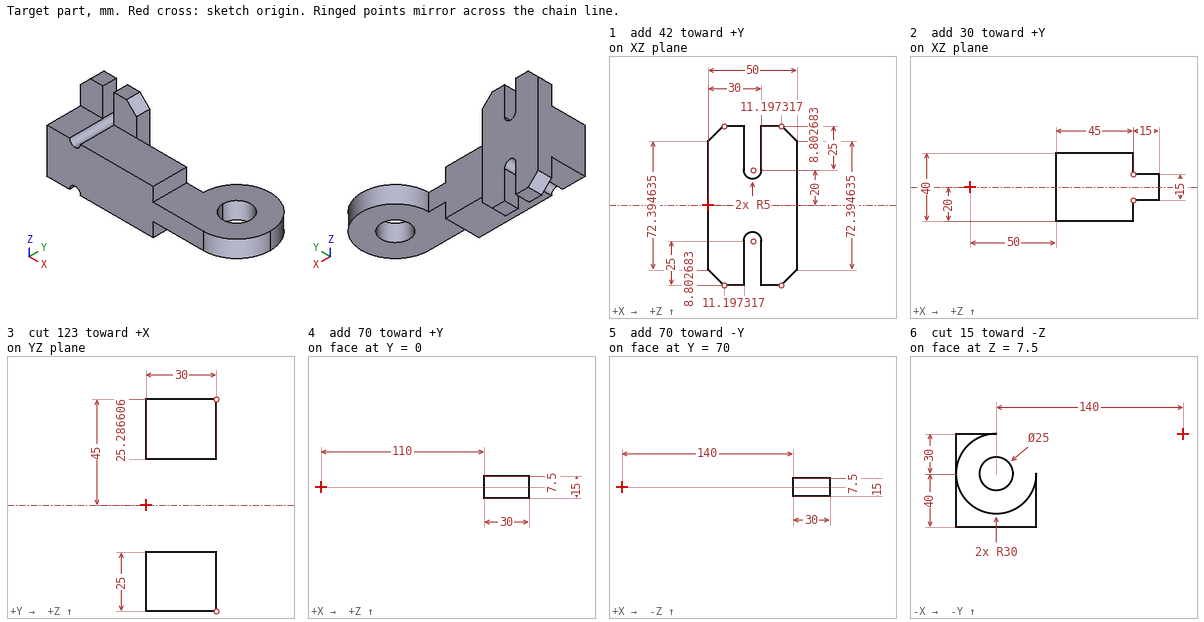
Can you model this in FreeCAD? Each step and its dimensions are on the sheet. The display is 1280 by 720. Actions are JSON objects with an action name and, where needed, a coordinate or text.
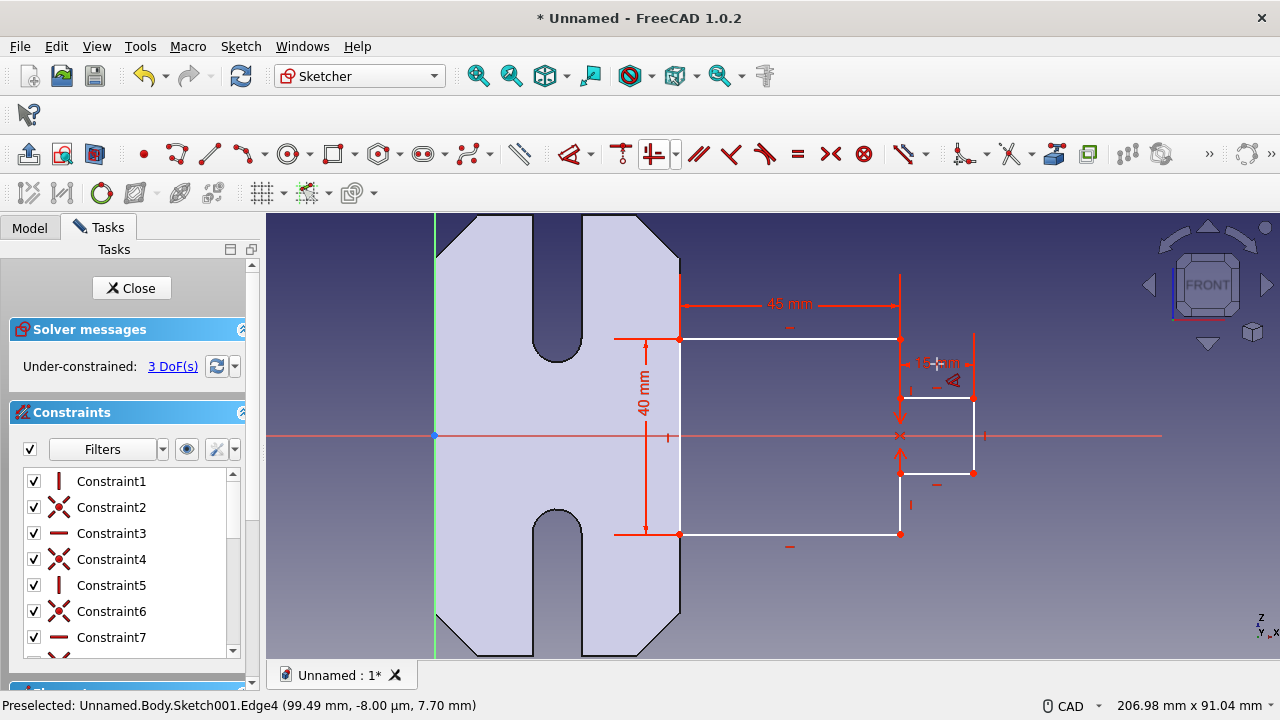
{"action": "left_click", "coordinate": [974, 421]}
{"action": "left_click", "coordinate": [1008, 419]}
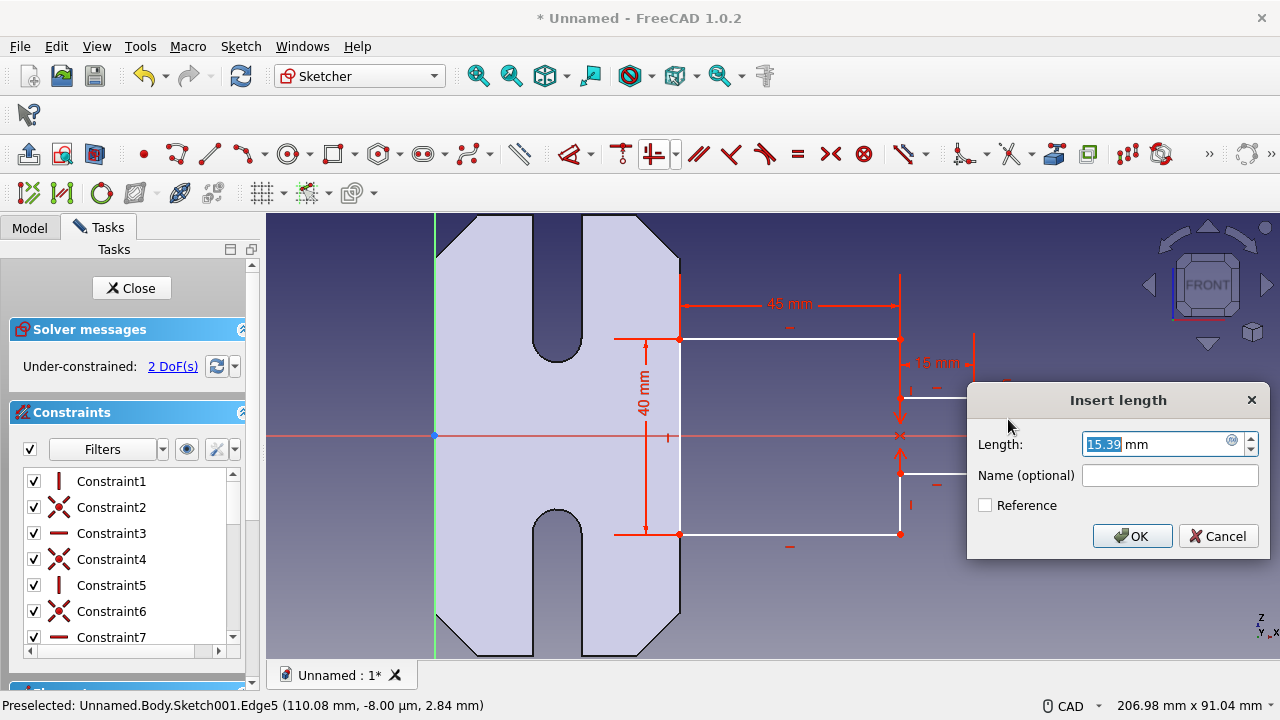
{"action": "type", "text": "15"}
{"action": "key", "text": "Return"}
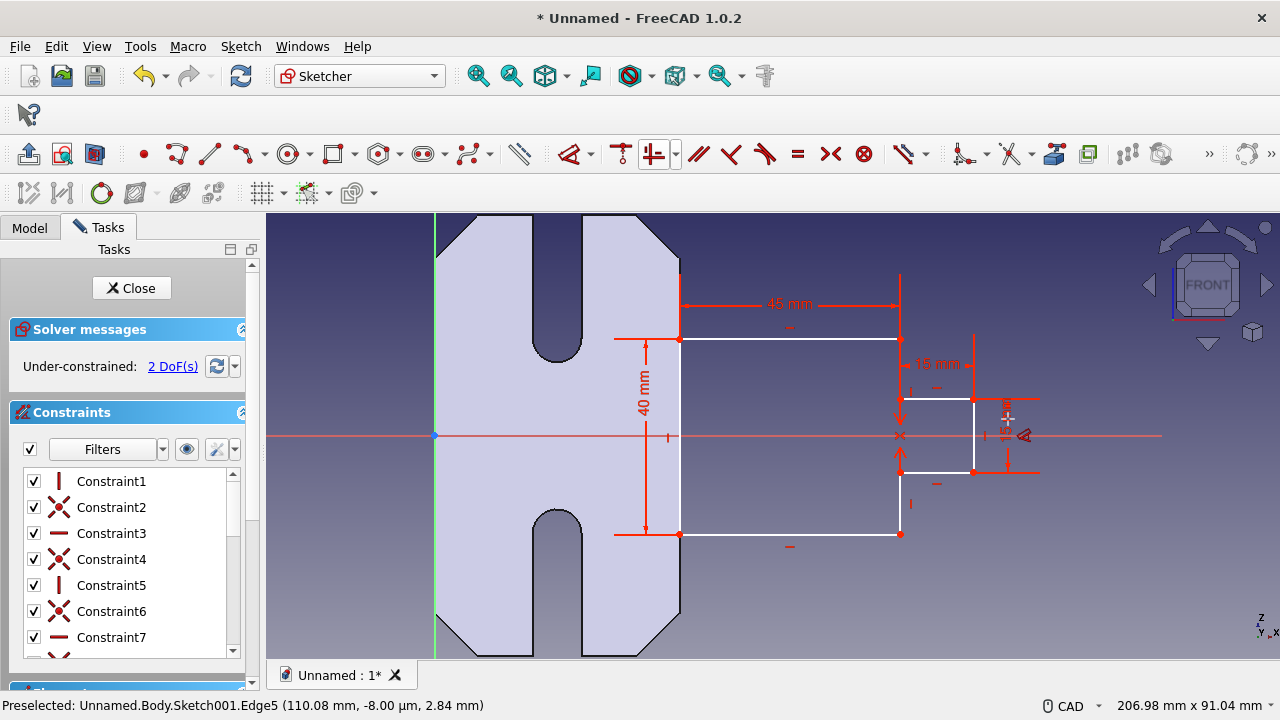
{"action": "left_click", "coordinate": [680, 535]}
{"action": "left_click", "coordinate": [557, 569]}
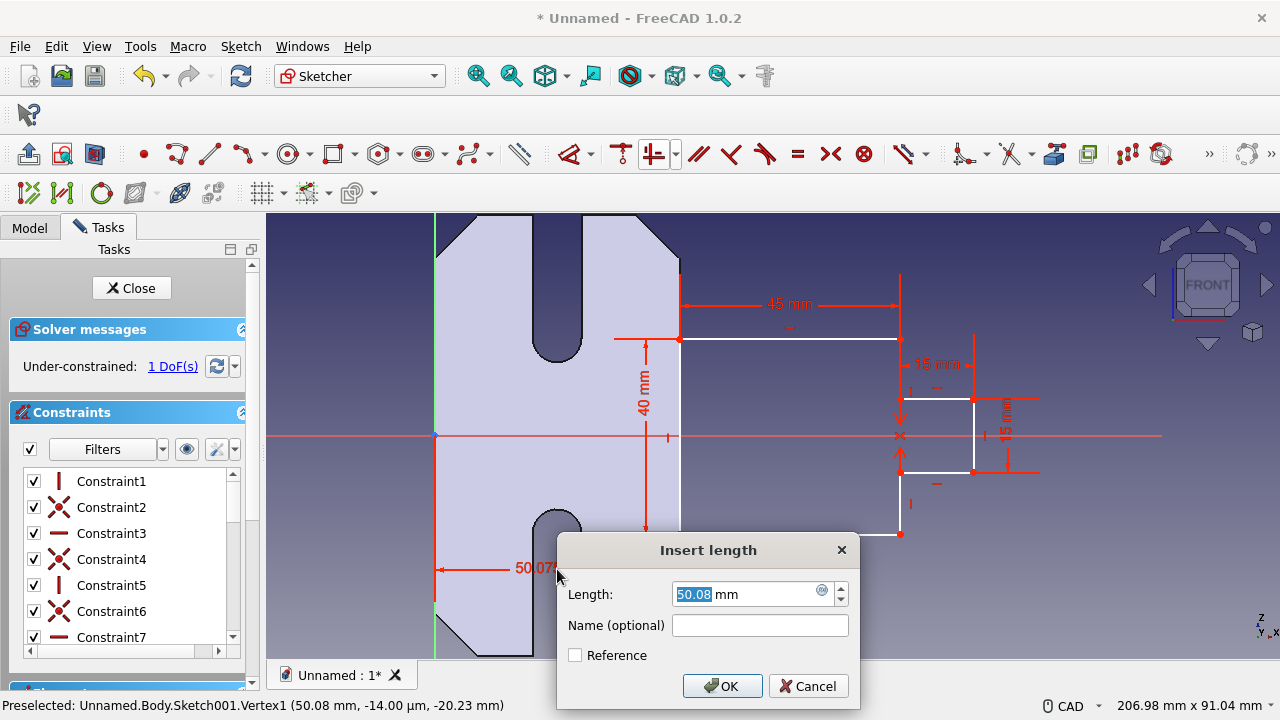
{"action": "type", "text": "50"}
{"action": "key", "text": "Return"}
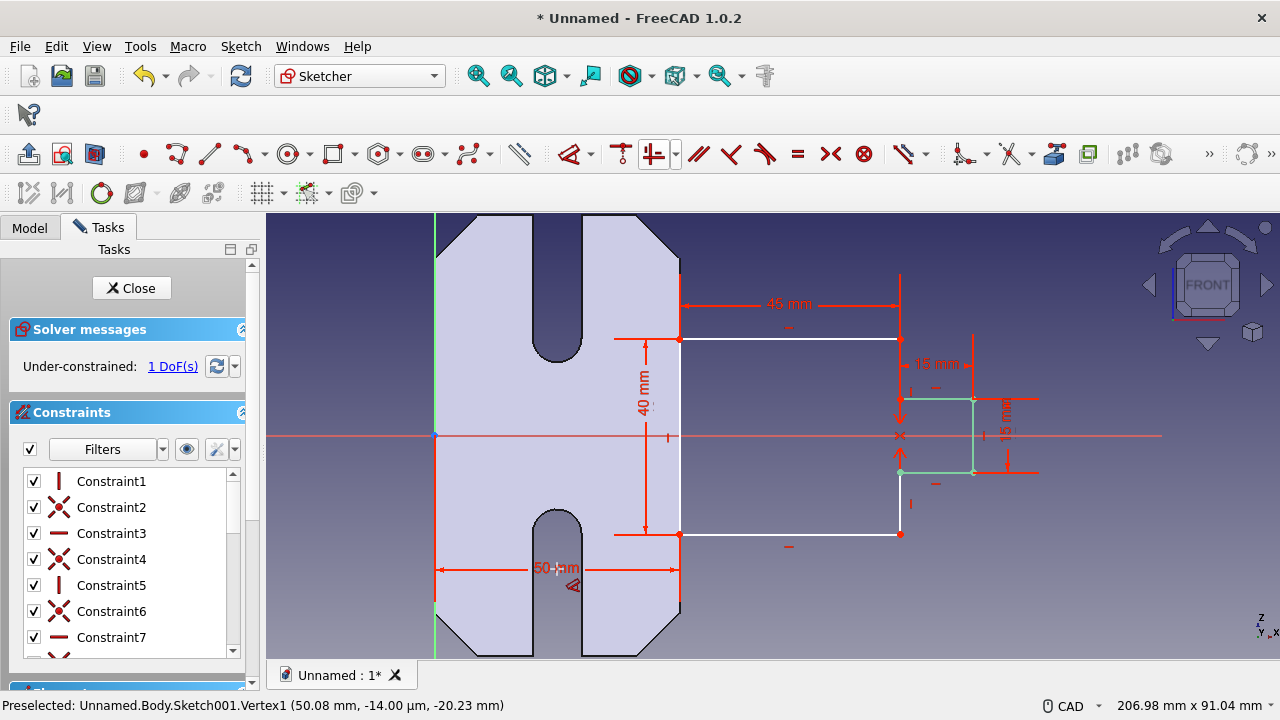
{"action": "left_click", "coordinate": [680, 535]}
{"action": "left_click", "coordinate": [401, 485]}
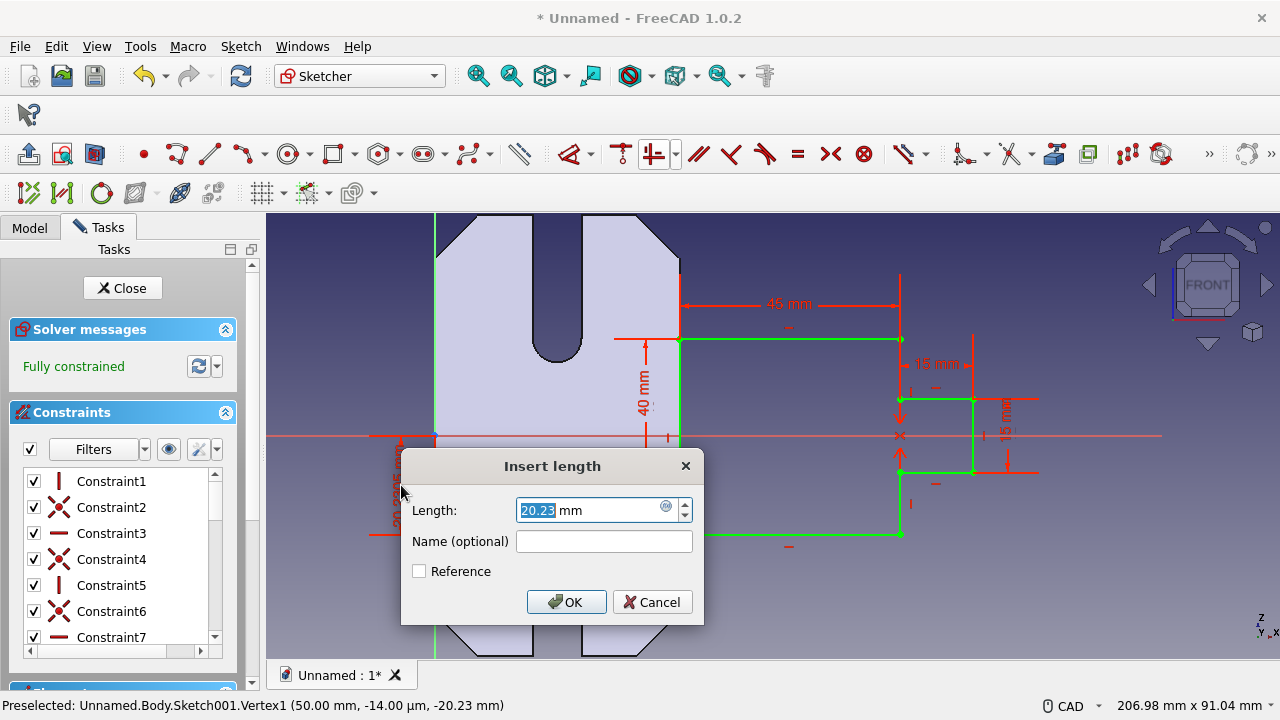
{"action": "type", "text": "20"}
{"action": "key", "text": "Return"}
{"action": "key", "text": "Escape"}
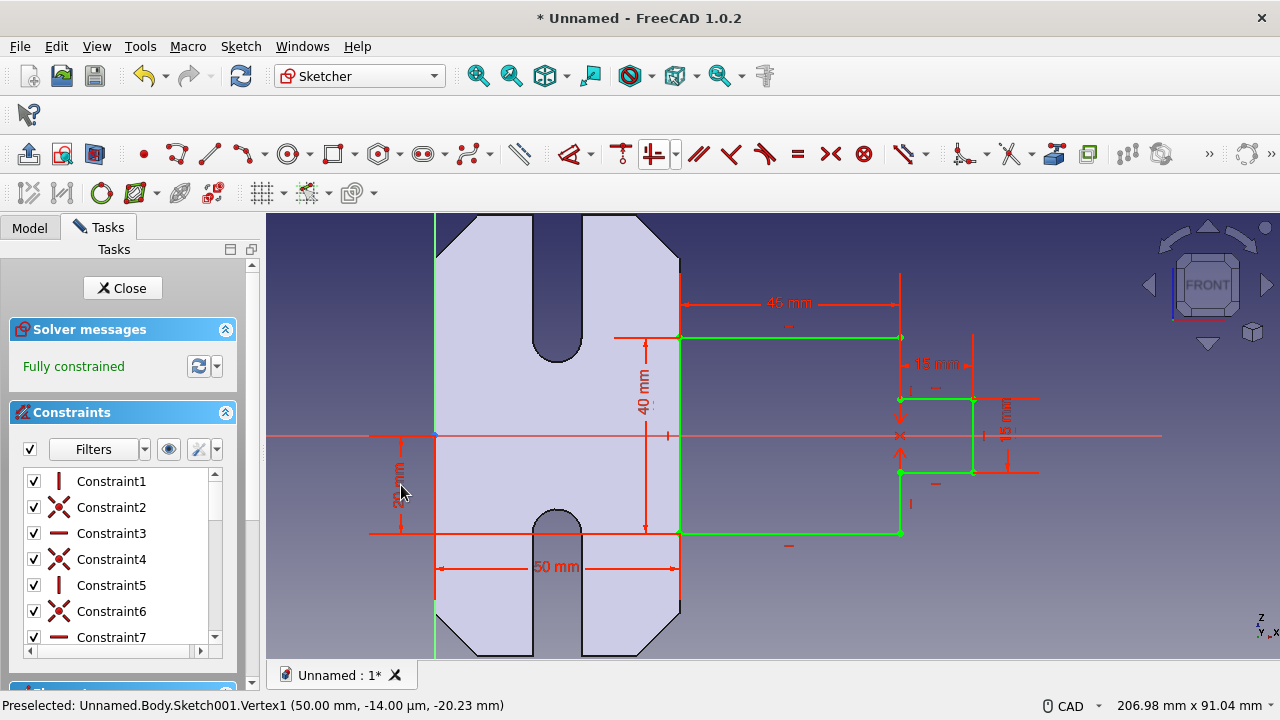
{"action": "left_click", "coordinate": [123, 288]}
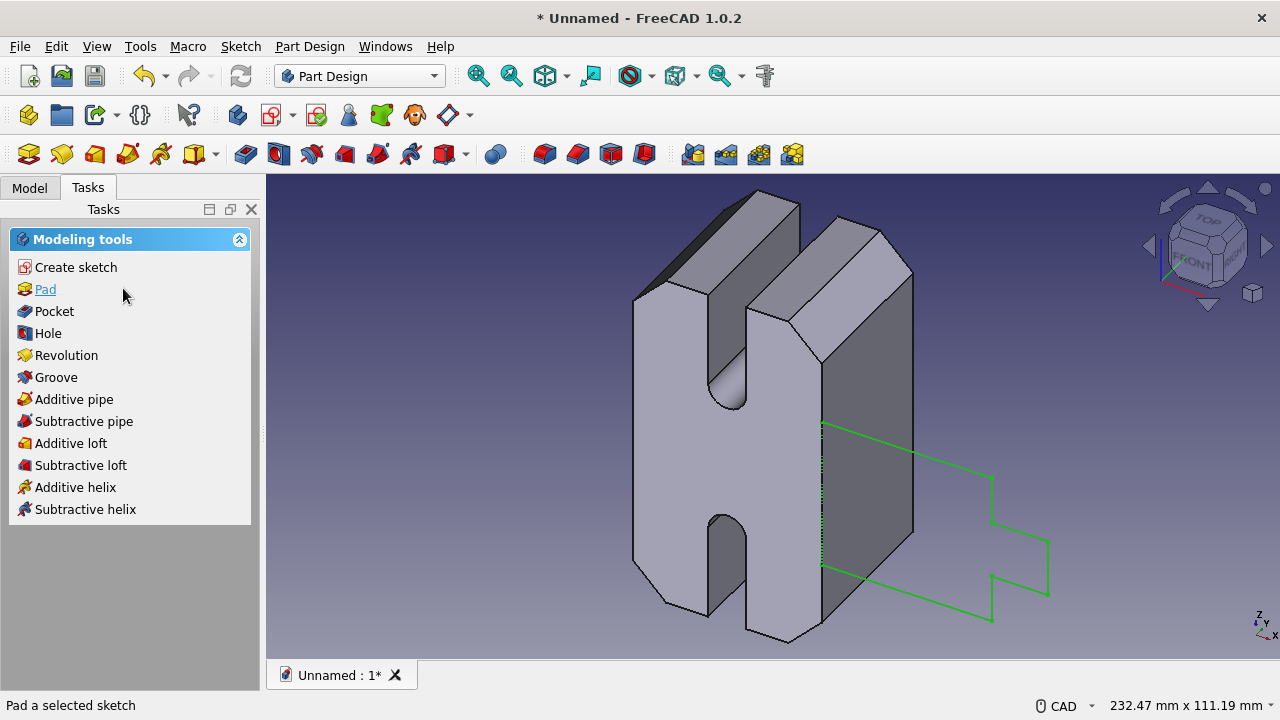
{"action": "left_click", "coordinate": [29, 154]}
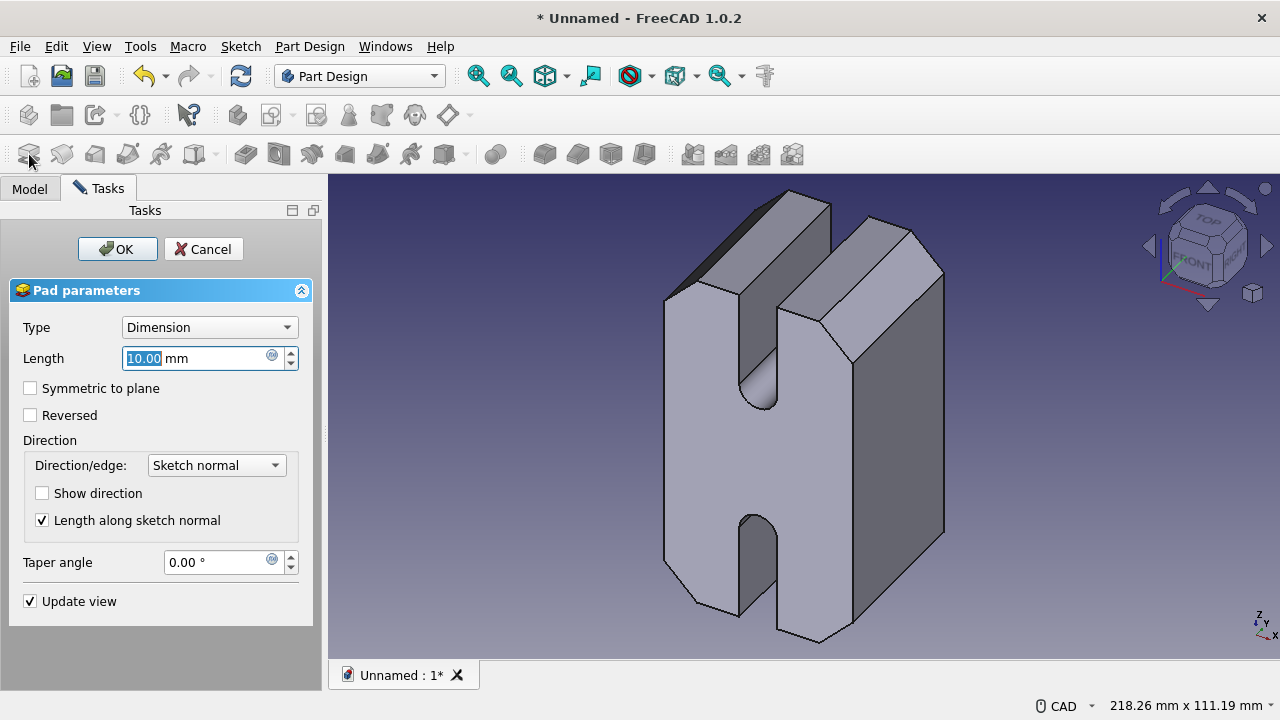
{"action": "type", "text": "30"}
{"action": "key", "text": "Tab"}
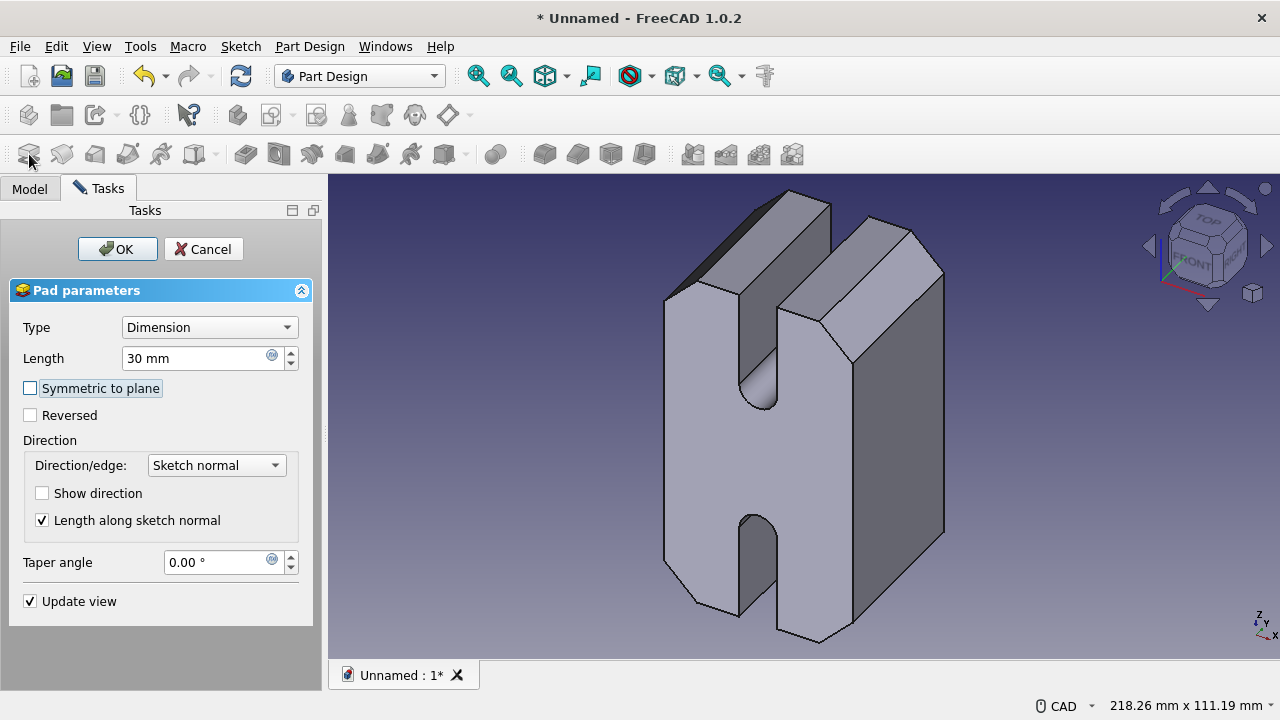
{"action": "left_click", "coordinate": [31, 415]}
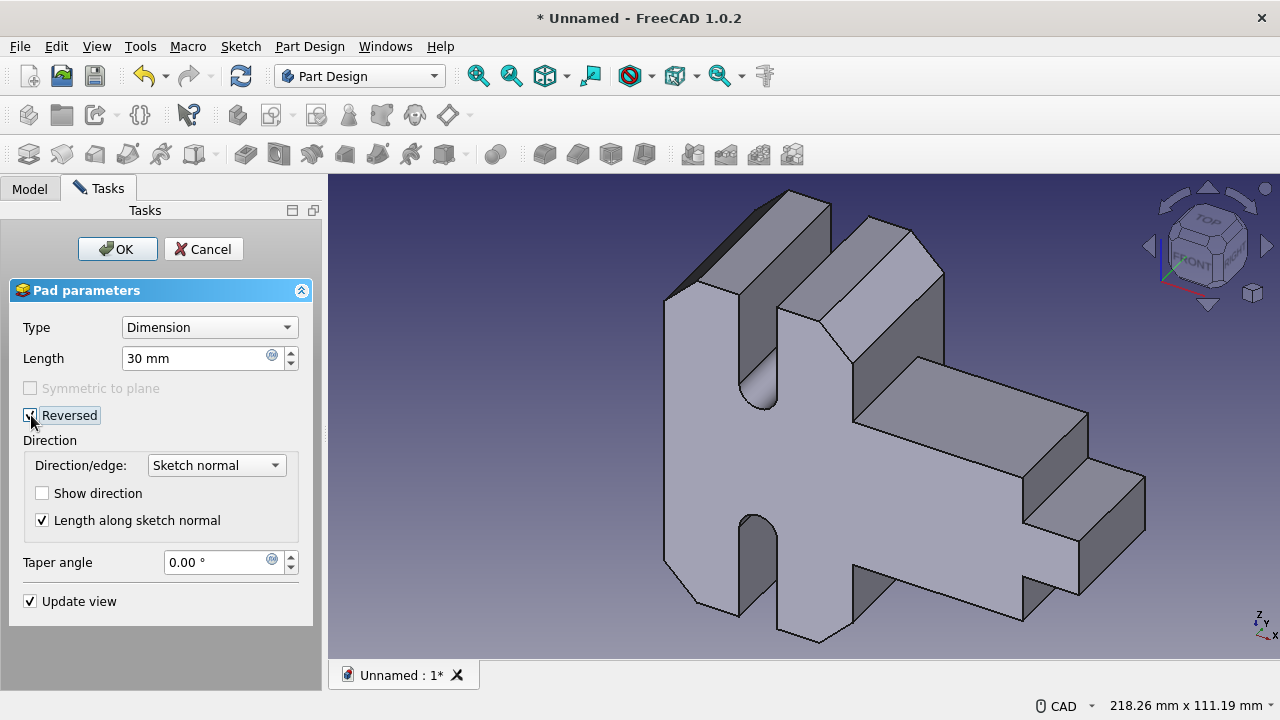
{"action": "left_click", "coordinate": [118, 249]}